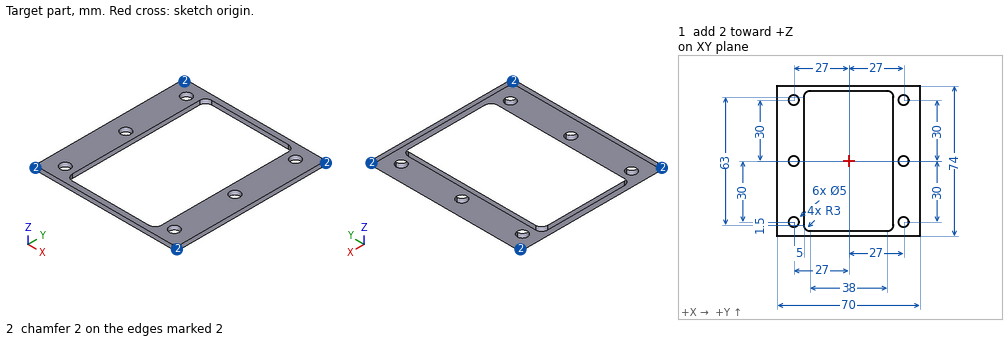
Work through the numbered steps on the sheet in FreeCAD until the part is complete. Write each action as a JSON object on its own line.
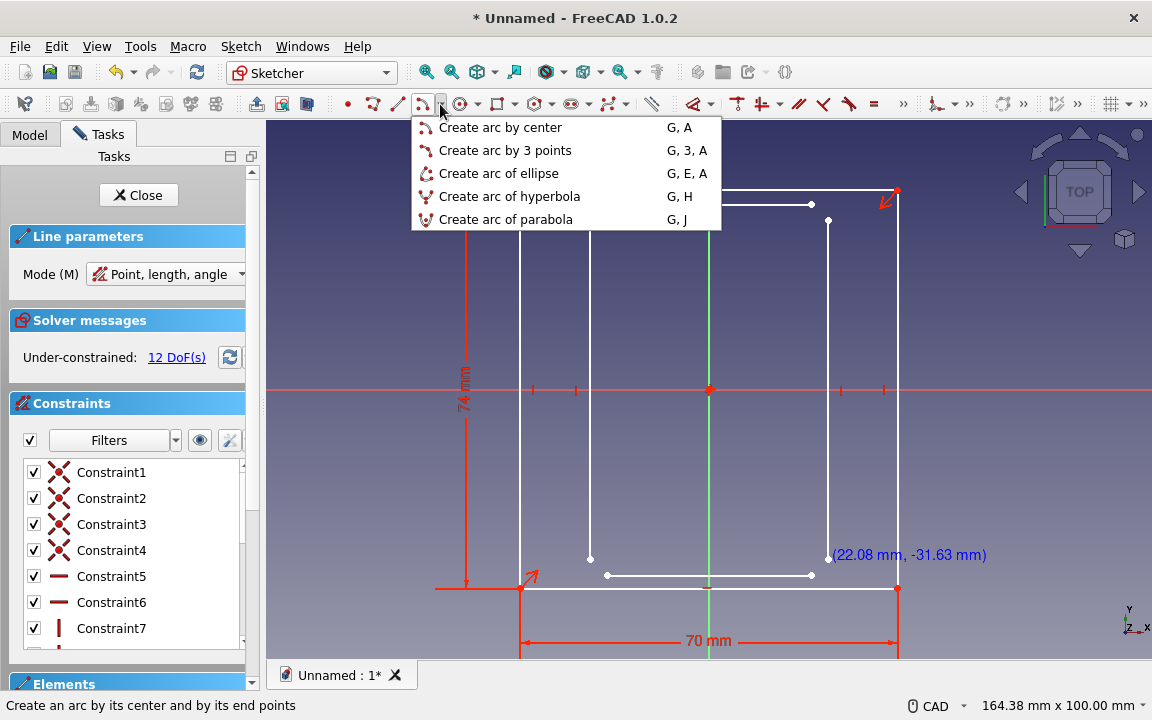
{"action": "left_click", "coordinate": [566, 150]}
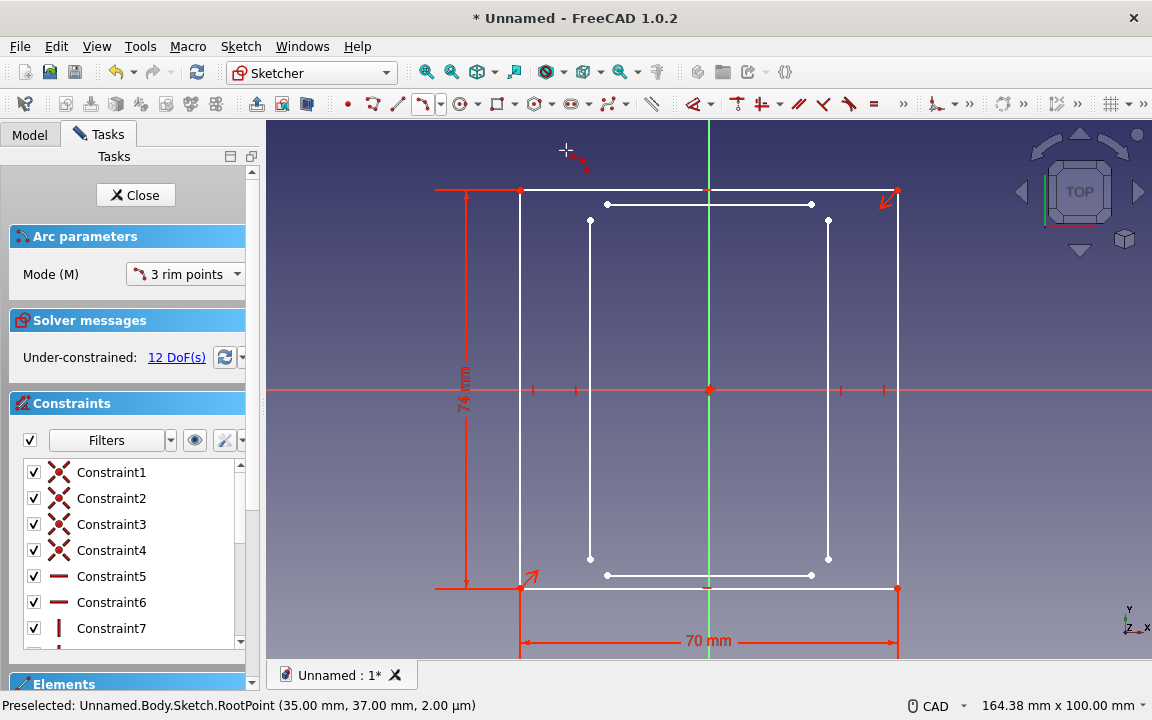
{"action": "left_click", "coordinate": [607, 576]}
{"action": "left_click", "coordinate": [590, 560]}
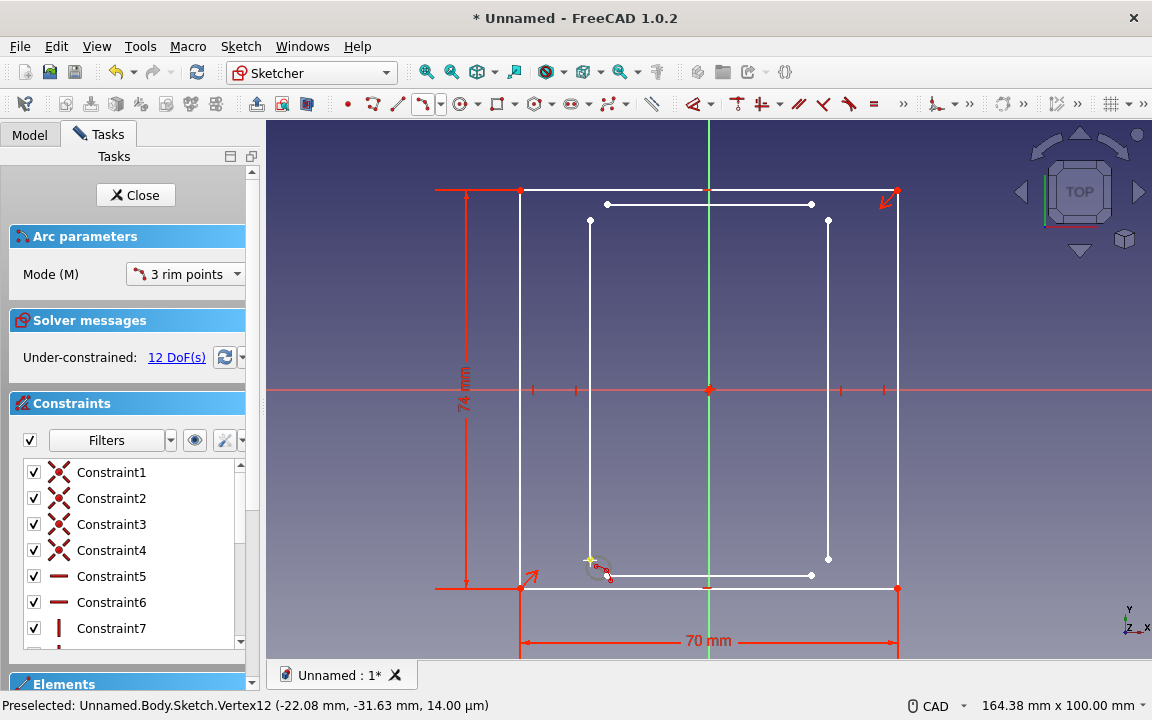
{"action": "scroll", "coordinate": [595, 571], "scroll_direction": "up", "scroll_amount": 7}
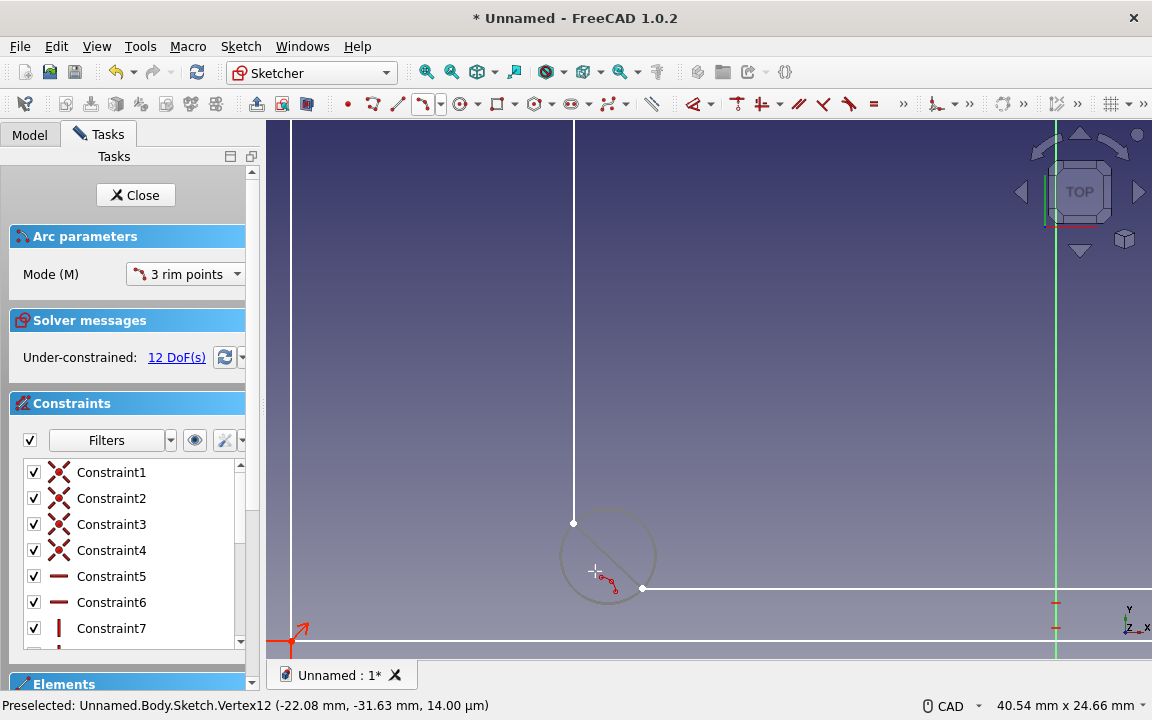
{"action": "left_click", "coordinate": [594, 567]}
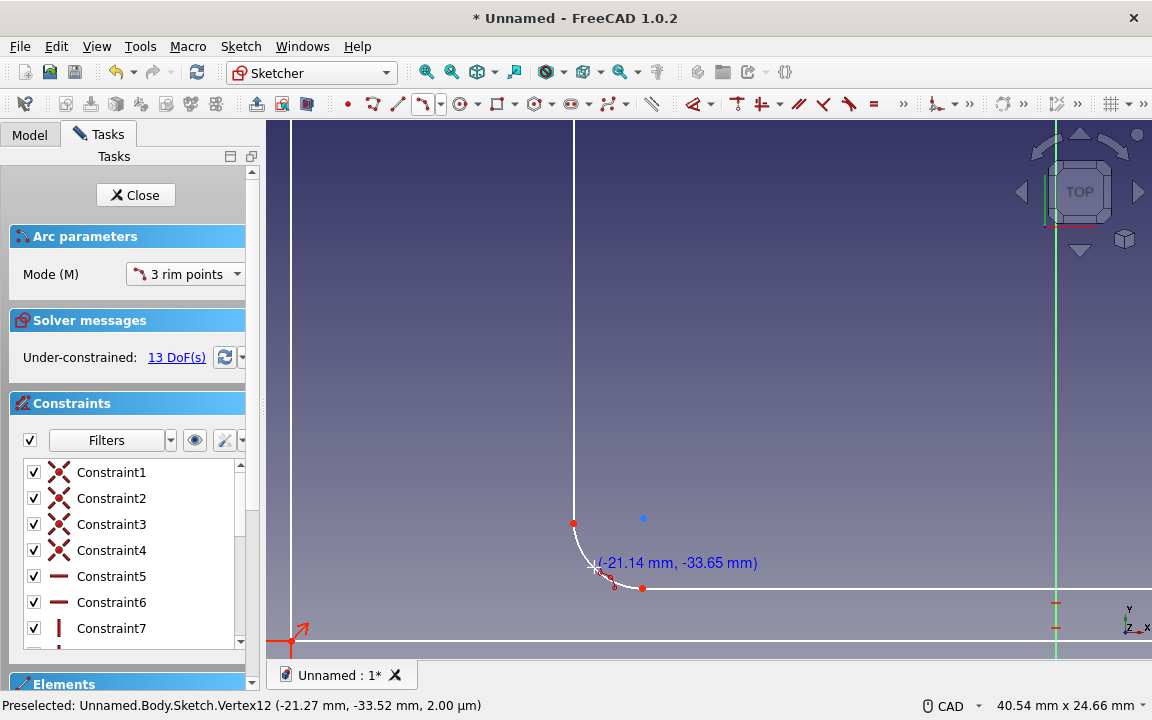
{"action": "scroll", "coordinate": [535, 530], "scroll_direction": "down", "scroll_amount": 8}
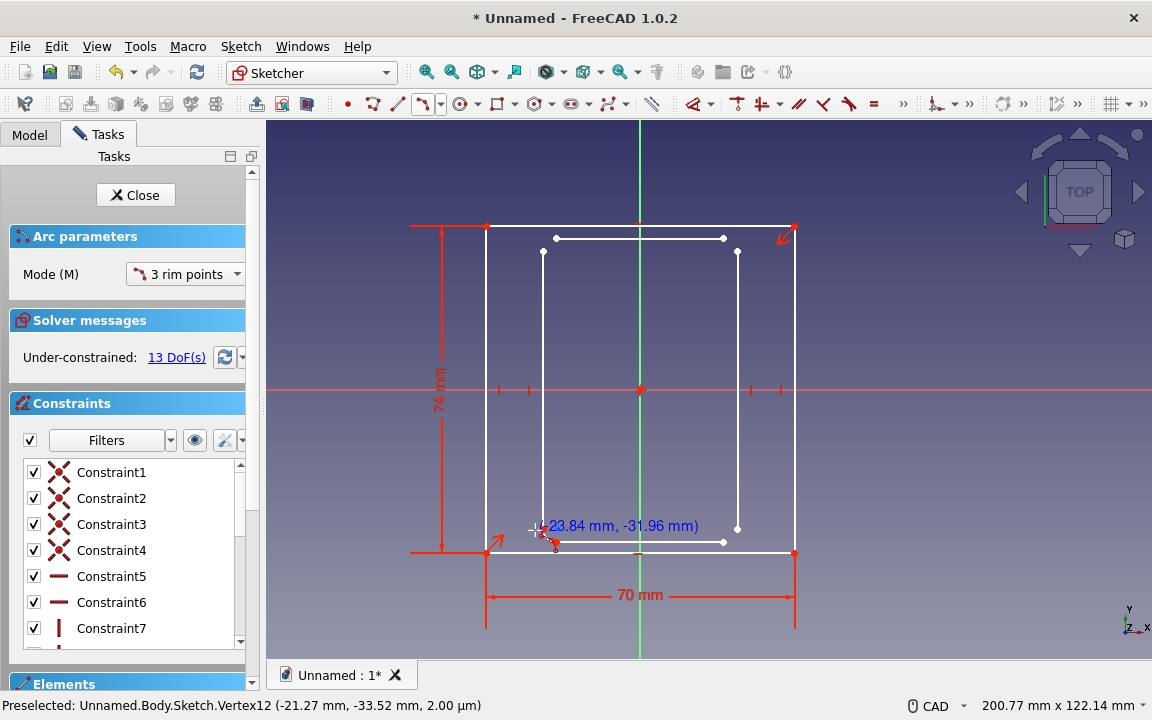
{"action": "left_click", "coordinate": [543, 252]}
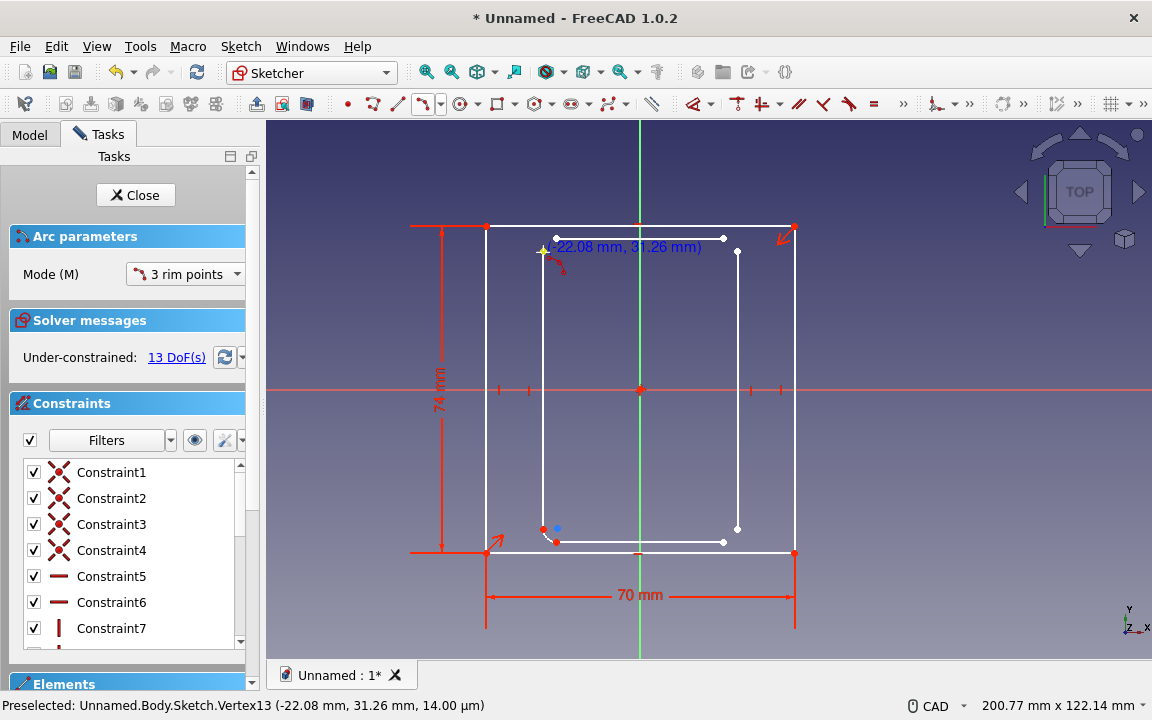
{"action": "scroll", "coordinate": [557, 238], "scroll_direction": "up", "scroll_amount": 2}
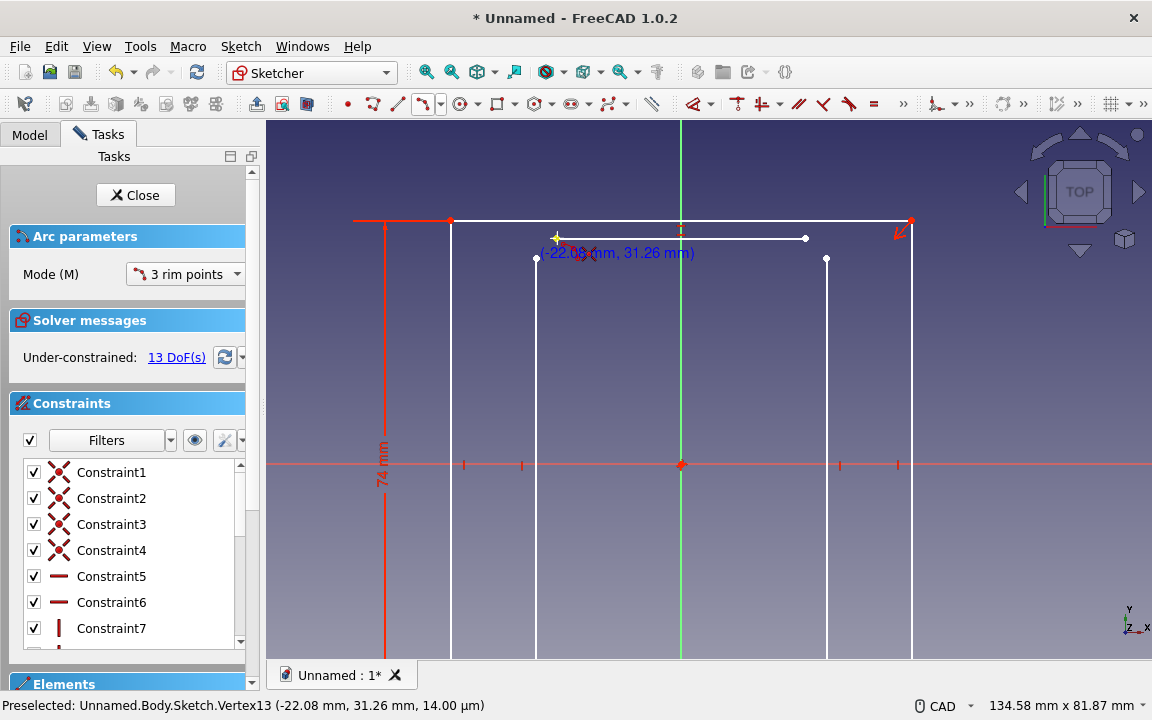
{"action": "left_click", "coordinate": [557, 239]}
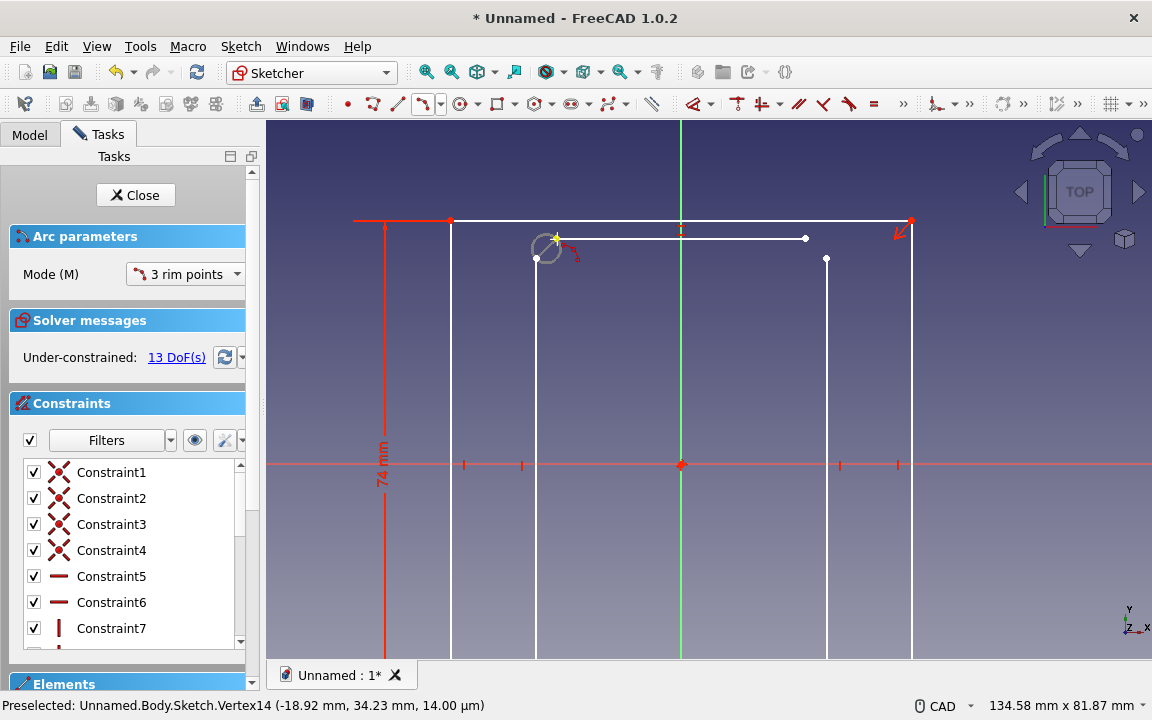
{"action": "scroll", "coordinate": [542, 243], "scroll_direction": "up", "scroll_amount": 6}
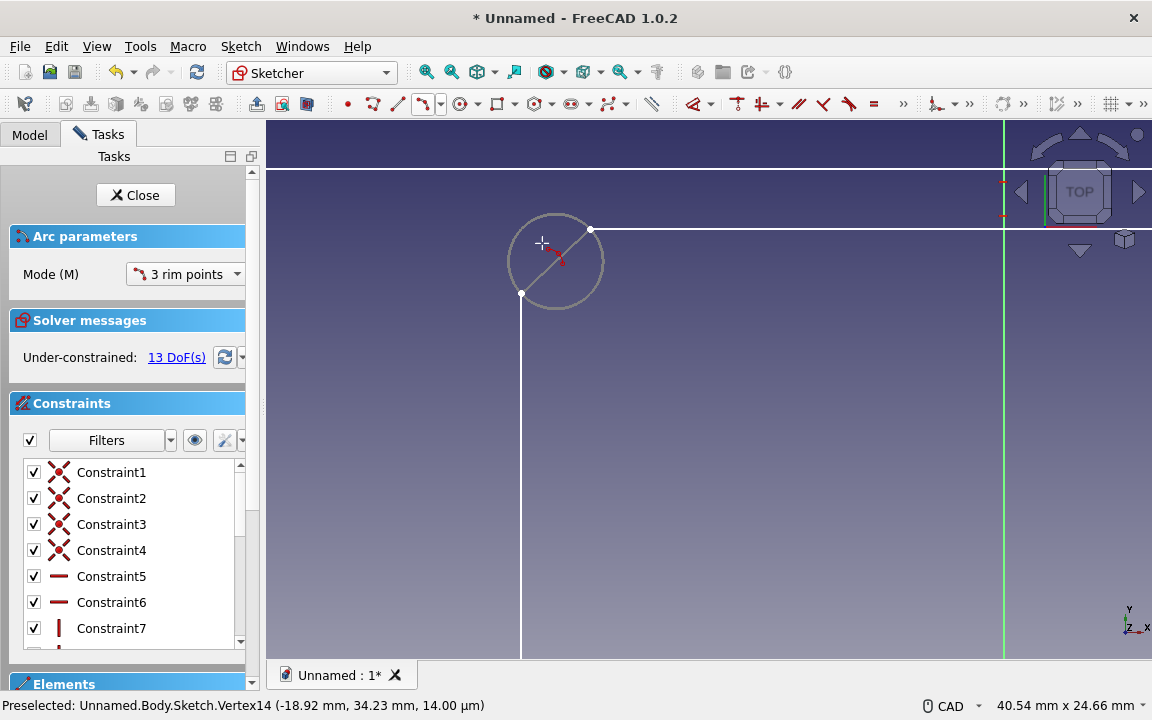
{"action": "left_click", "coordinate": [542, 242]}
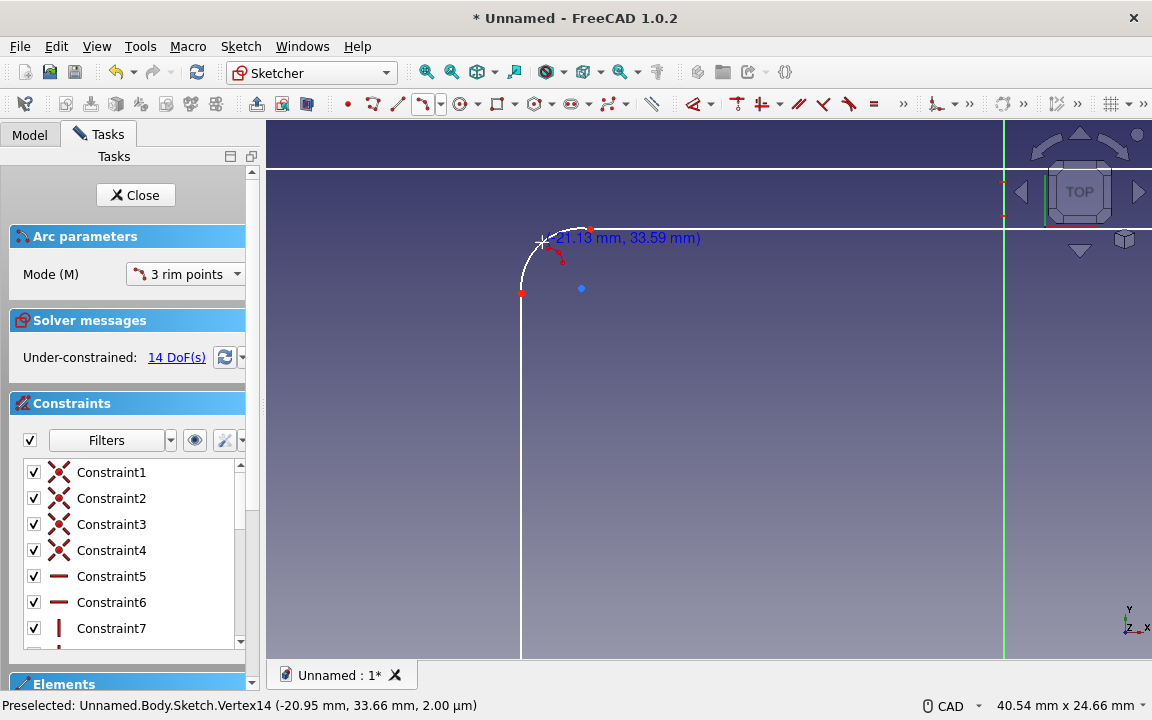
{"action": "scroll", "coordinate": [549, 241], "scroll_direction": "down", "scroll_amount": 8}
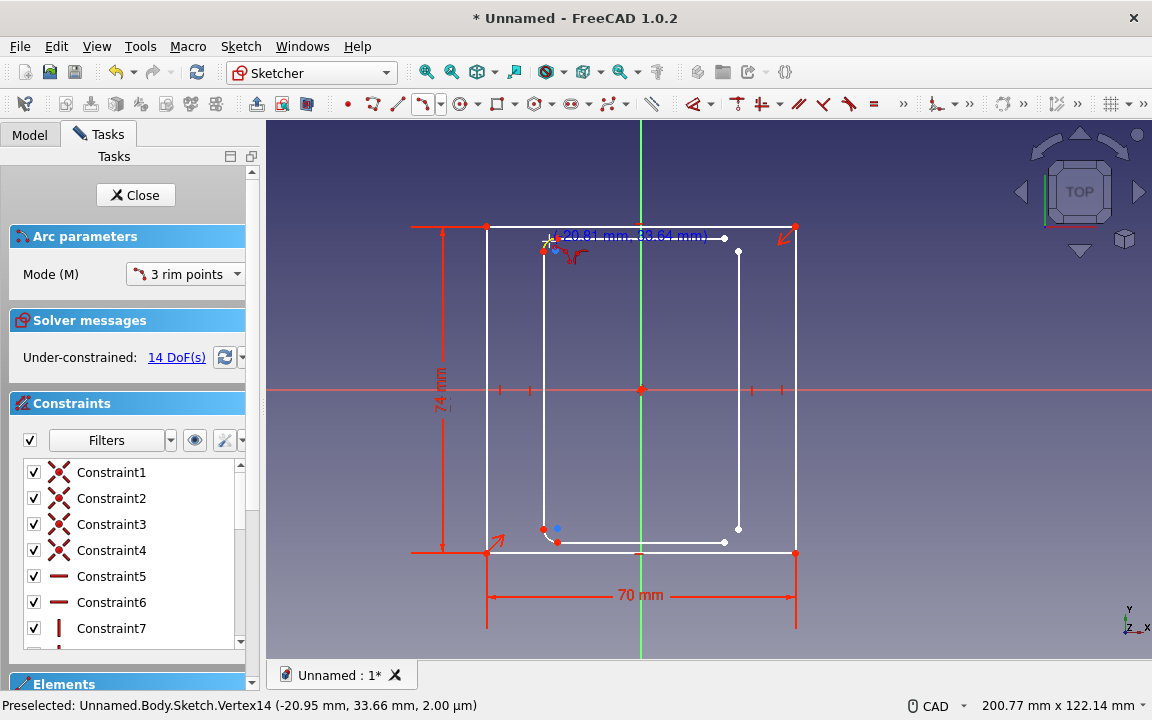
{"action": "scroll", "coordinate": [725, 238], "scroll_direction": "up", "scroll_amount": 2}